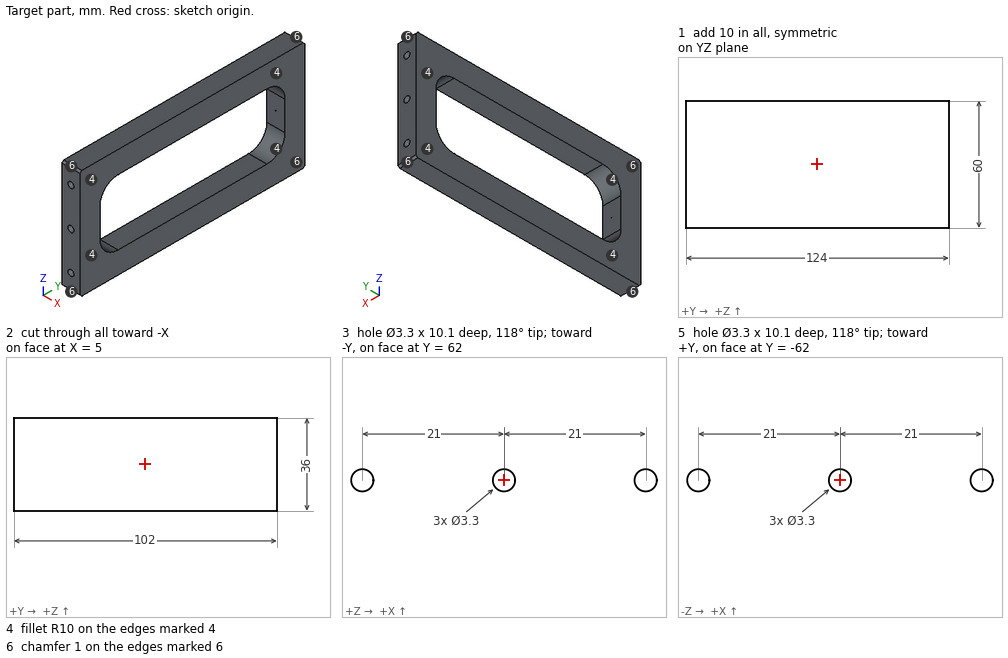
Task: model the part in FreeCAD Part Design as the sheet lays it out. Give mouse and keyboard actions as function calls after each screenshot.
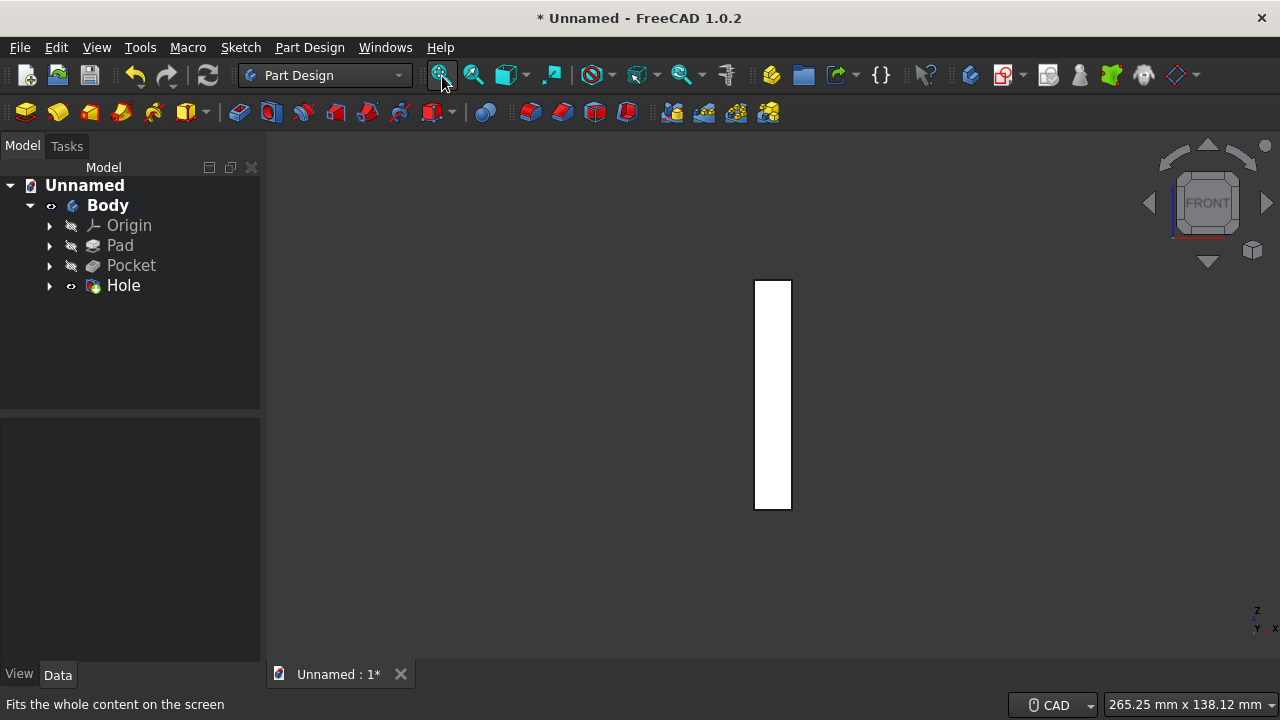
key(3)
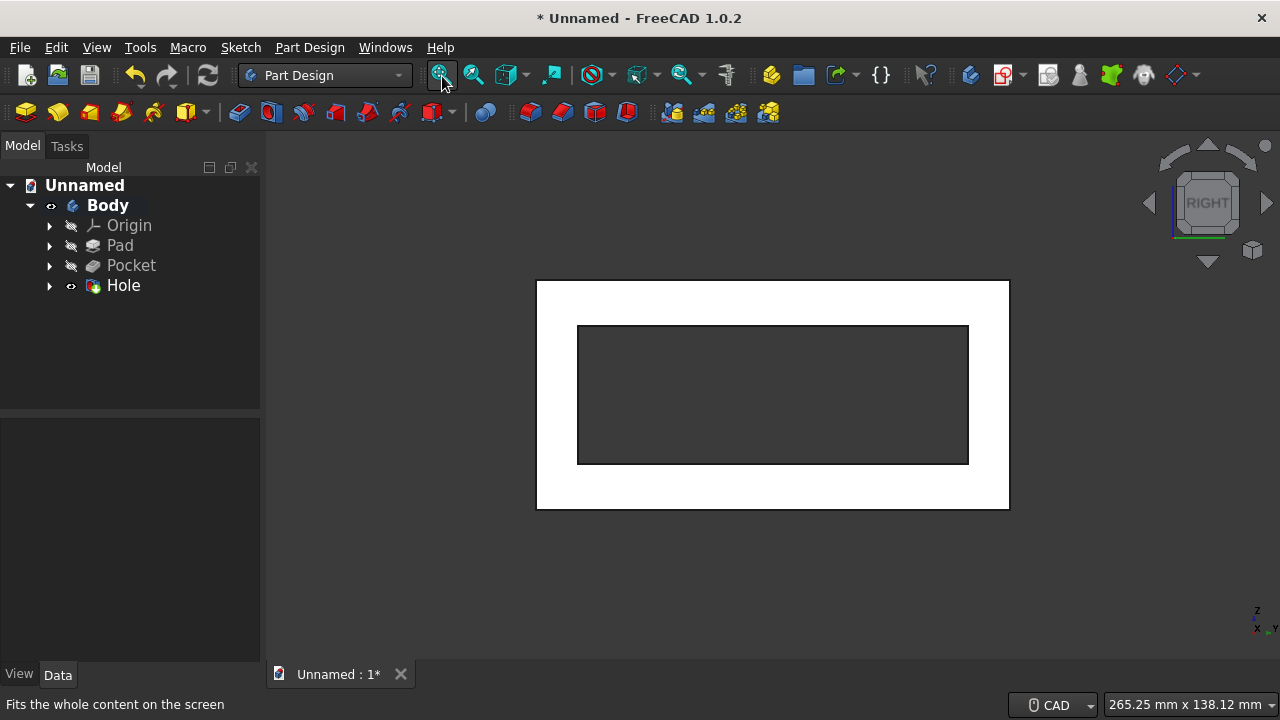
key(5)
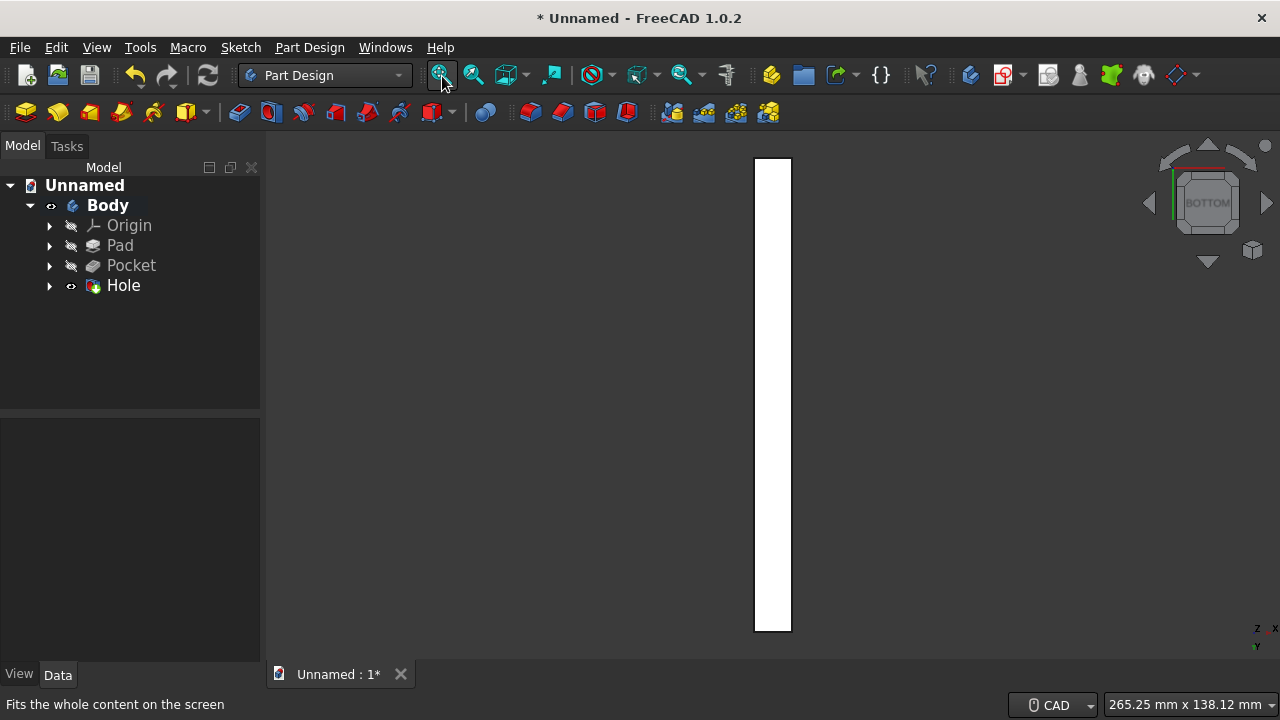
key(4)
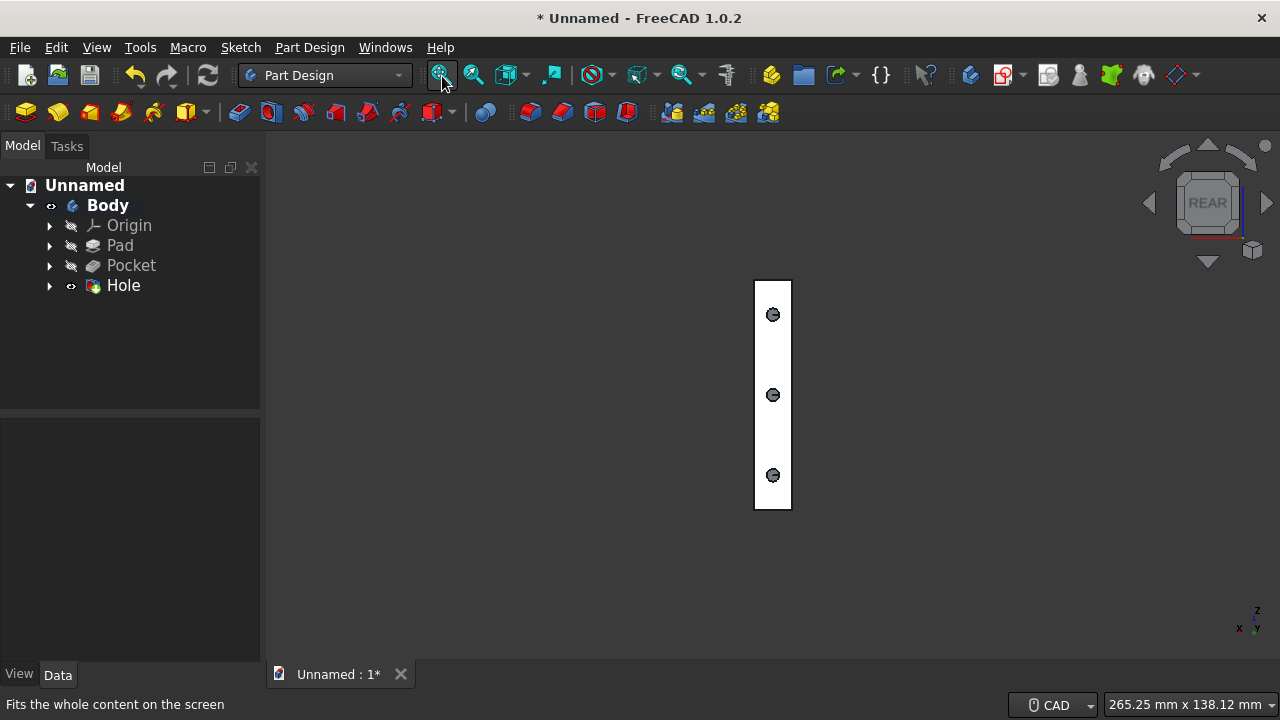
click(442, 76)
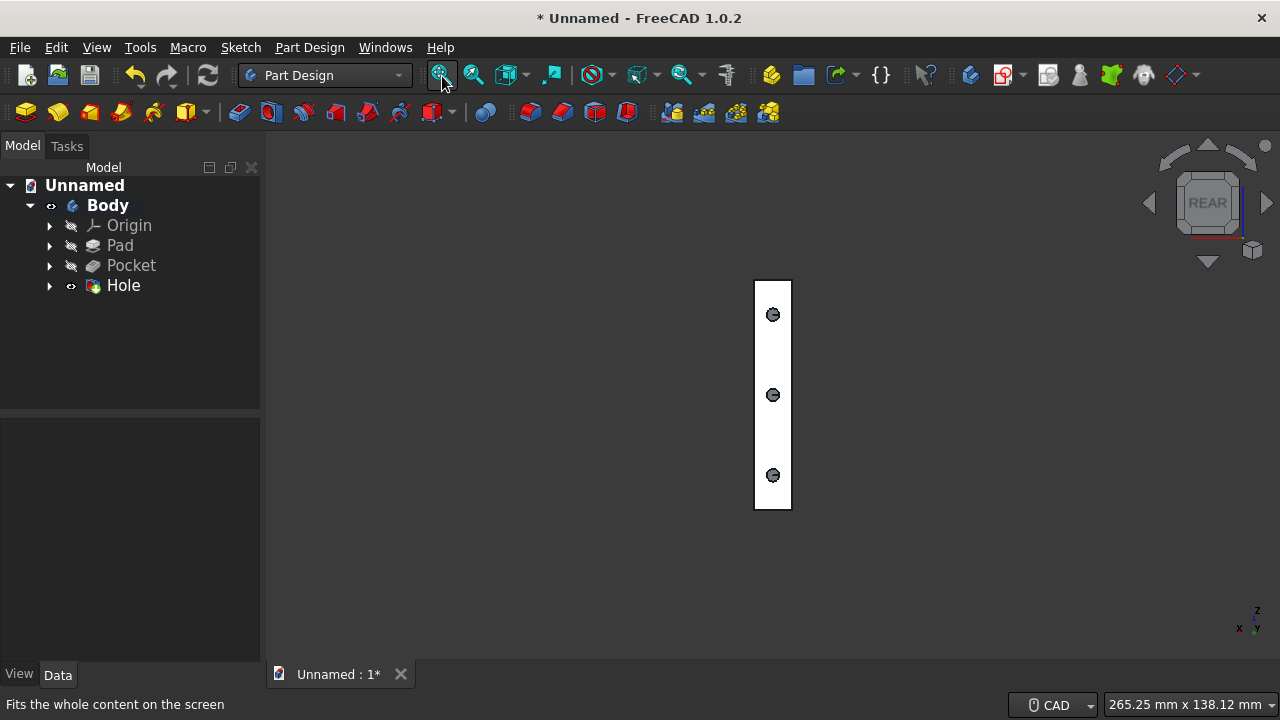
key(6)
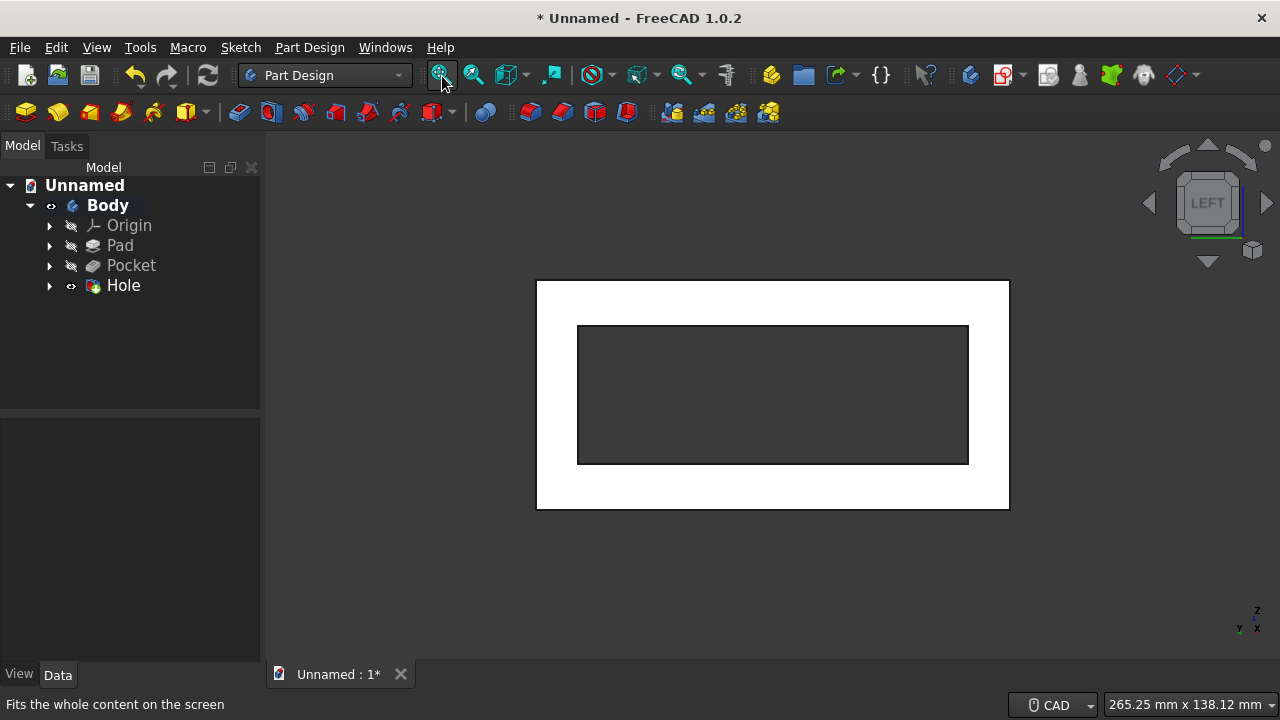
key(v)
key(3)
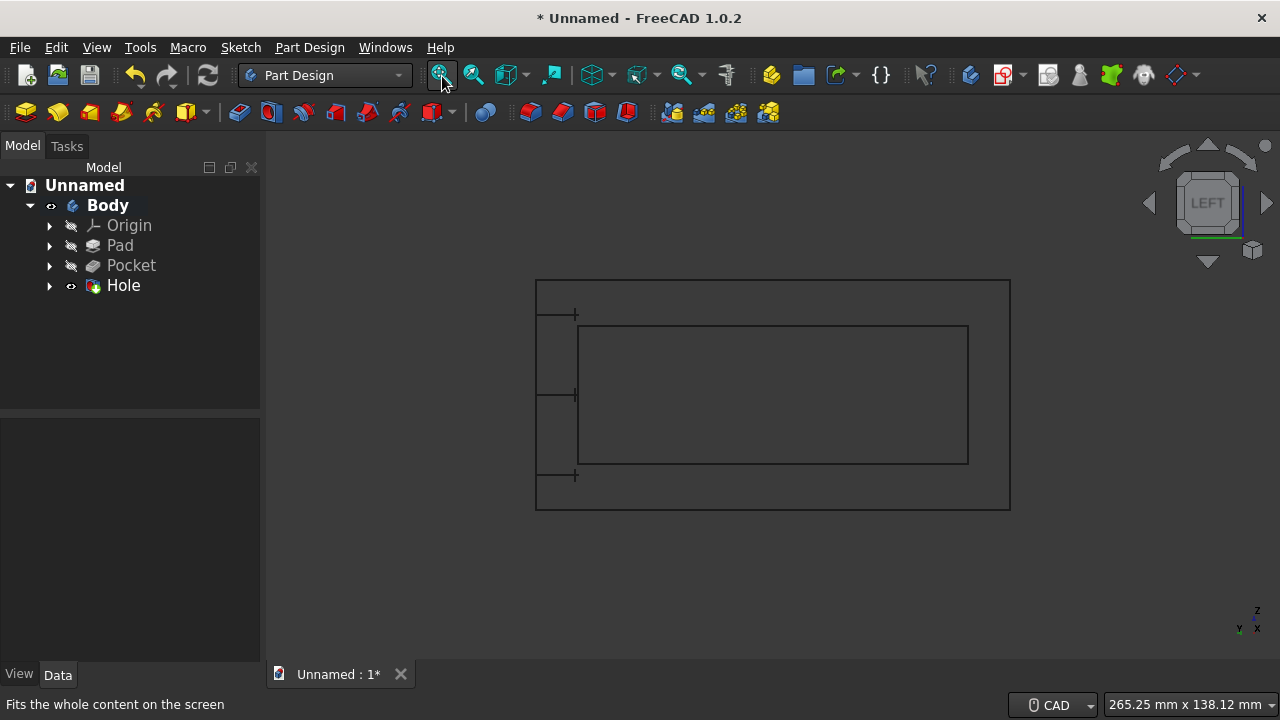
key(0)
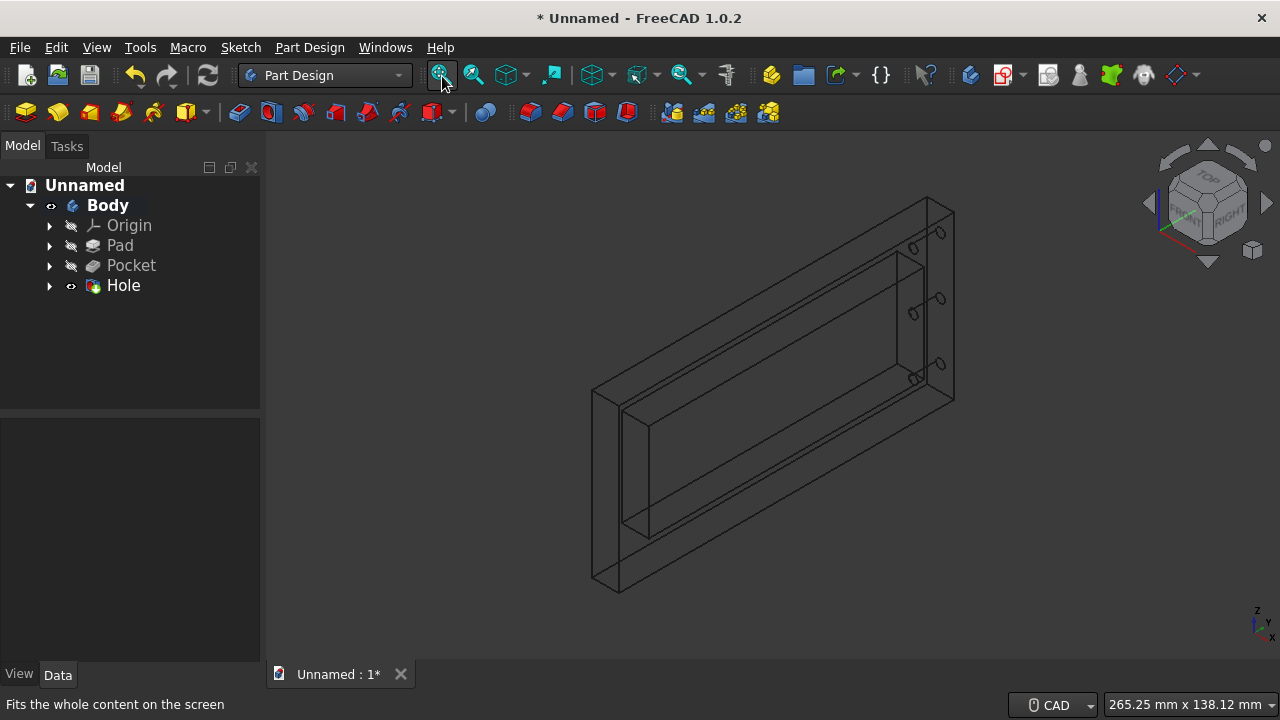
click(911, 371)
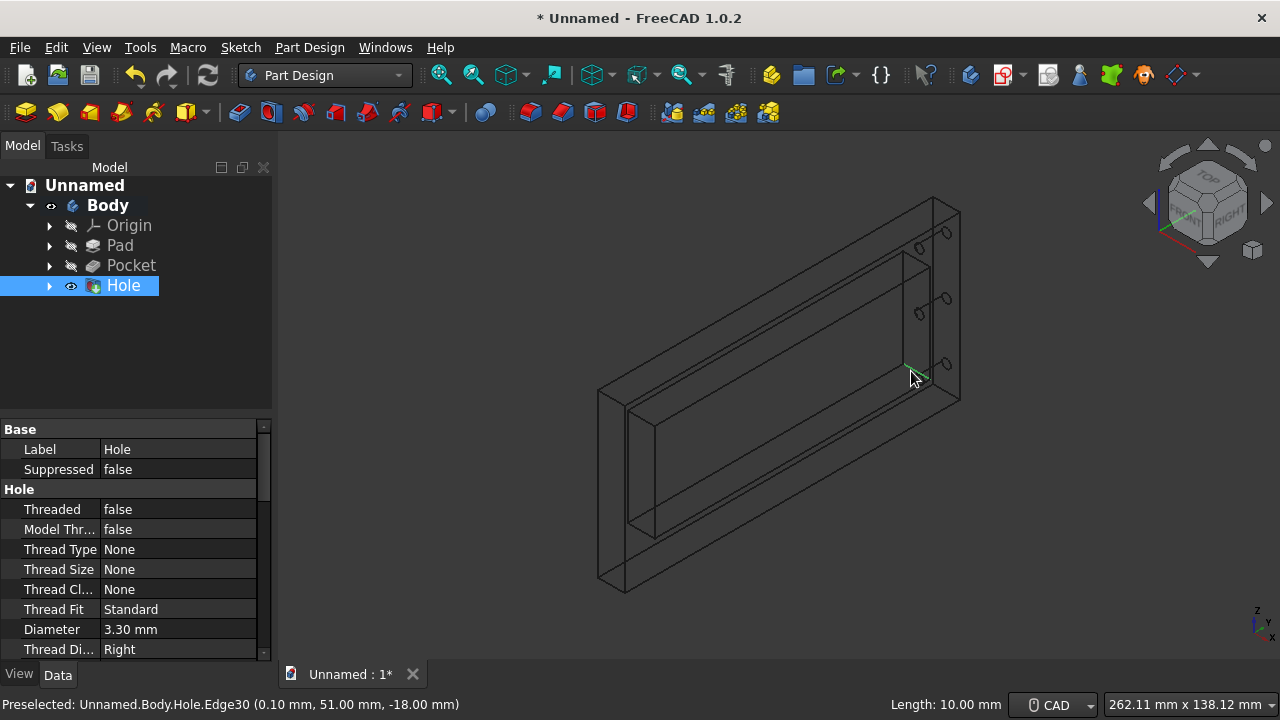
click(641, 530, ctrl)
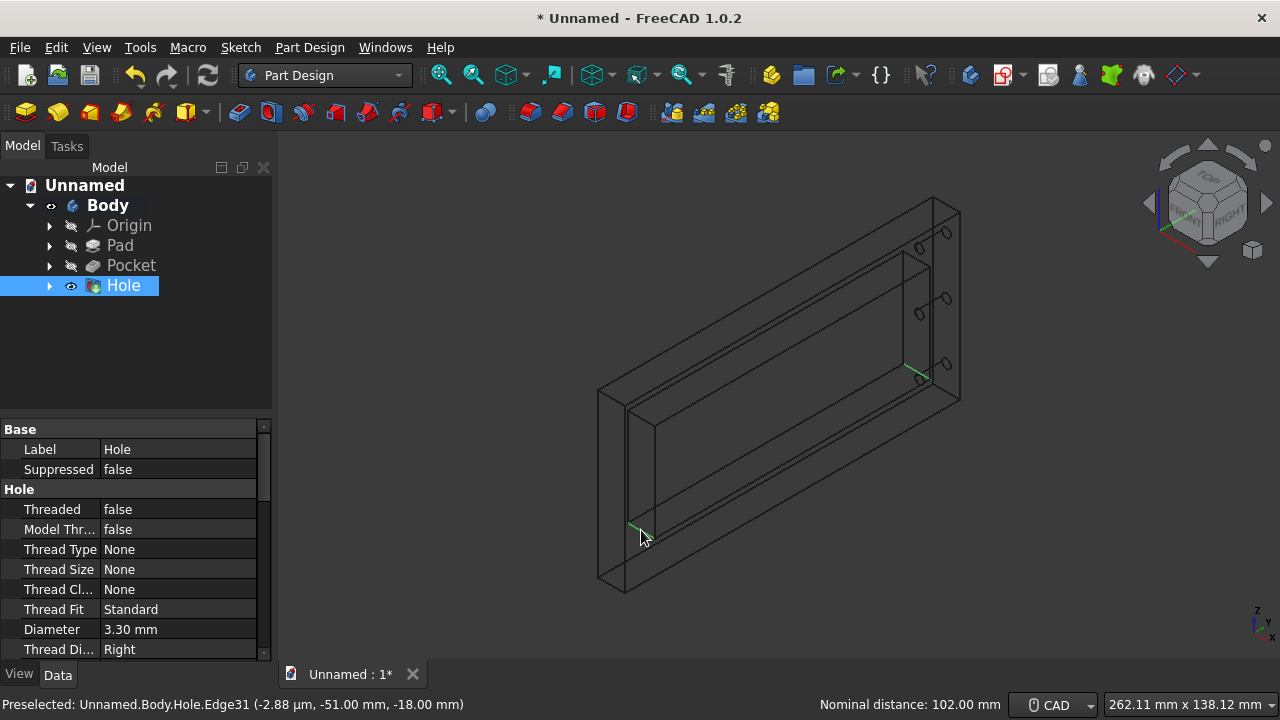
click(641, 417, ctrl)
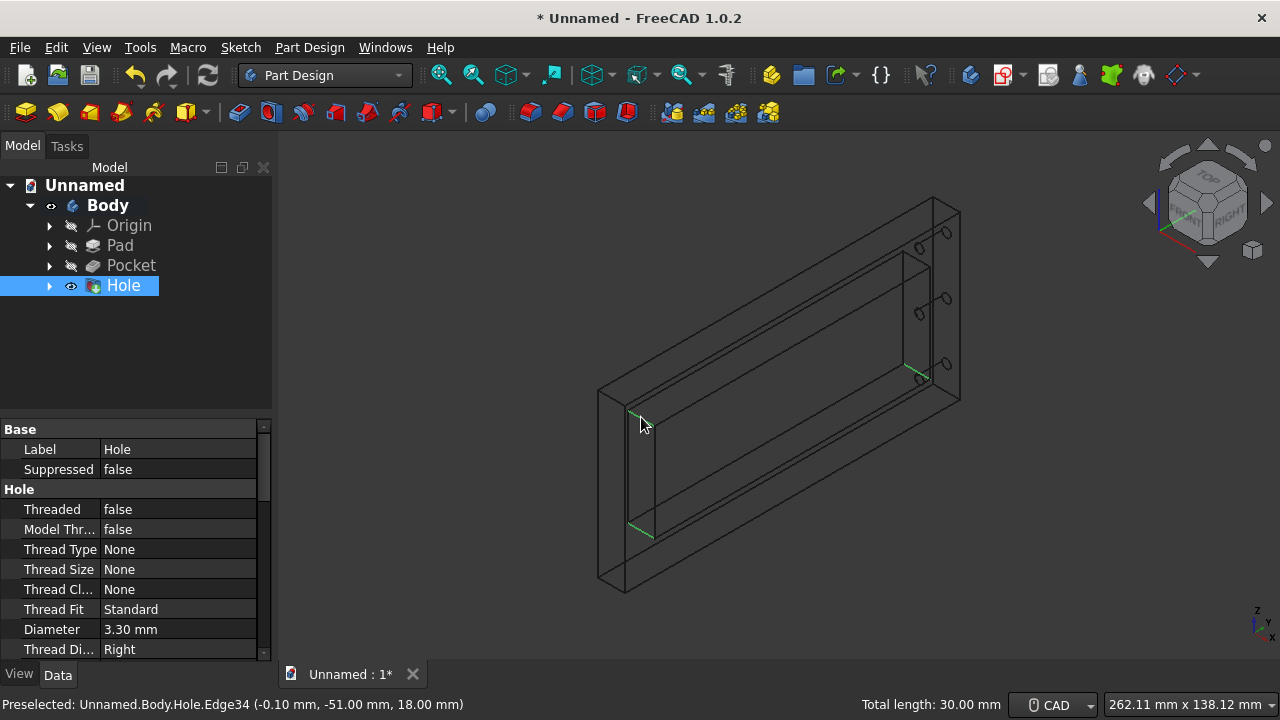
click(920, 260, ctrl)